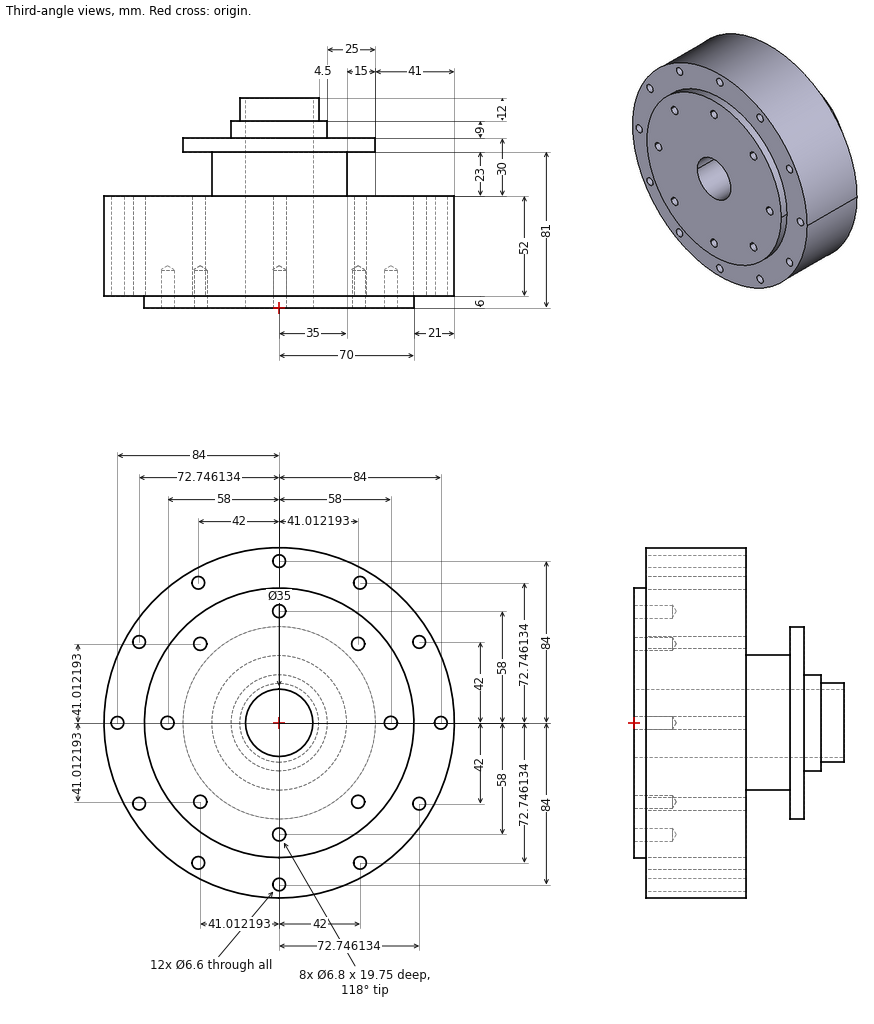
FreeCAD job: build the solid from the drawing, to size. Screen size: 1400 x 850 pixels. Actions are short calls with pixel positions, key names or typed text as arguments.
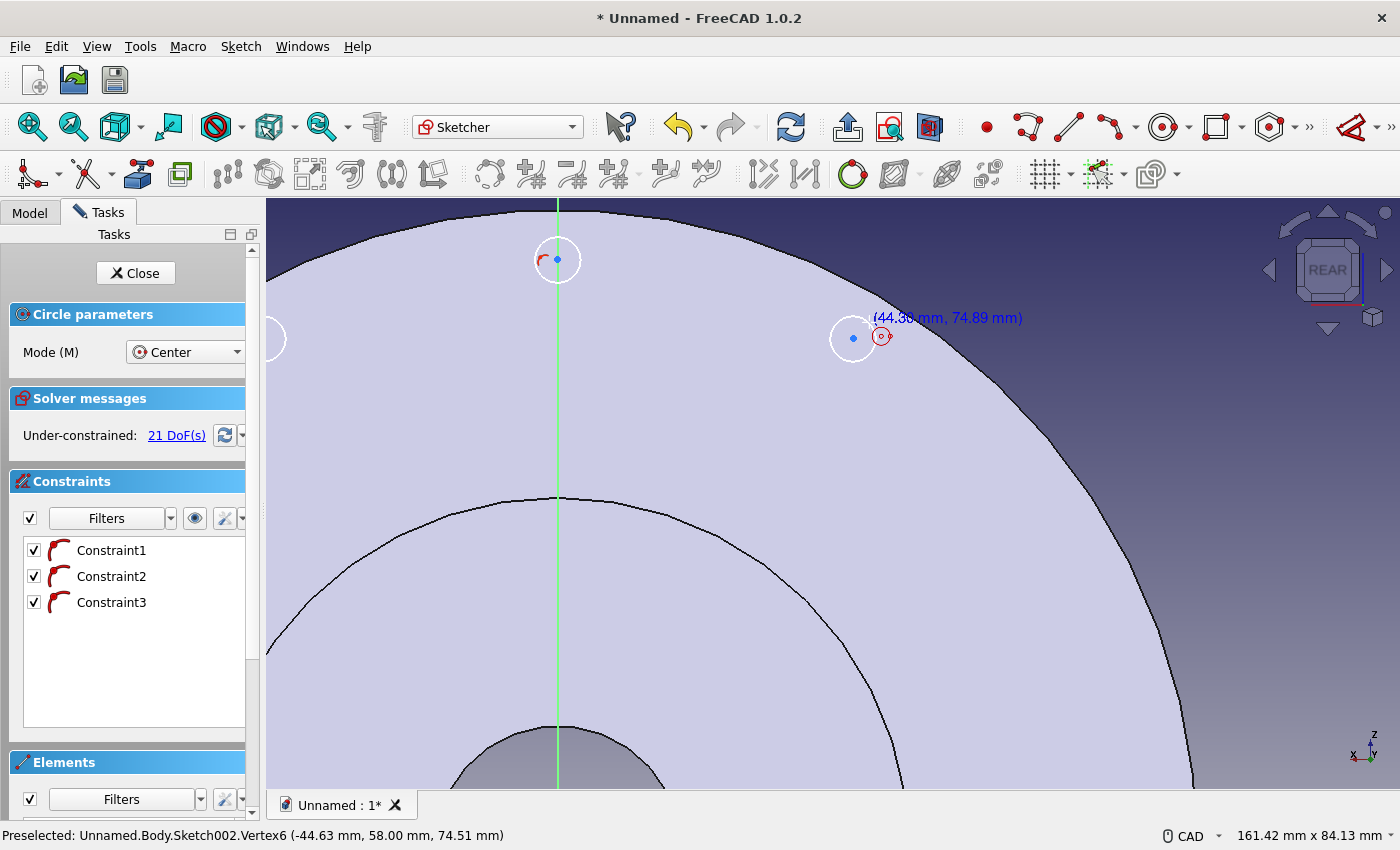
click(1069, 554)
click(1085, 538)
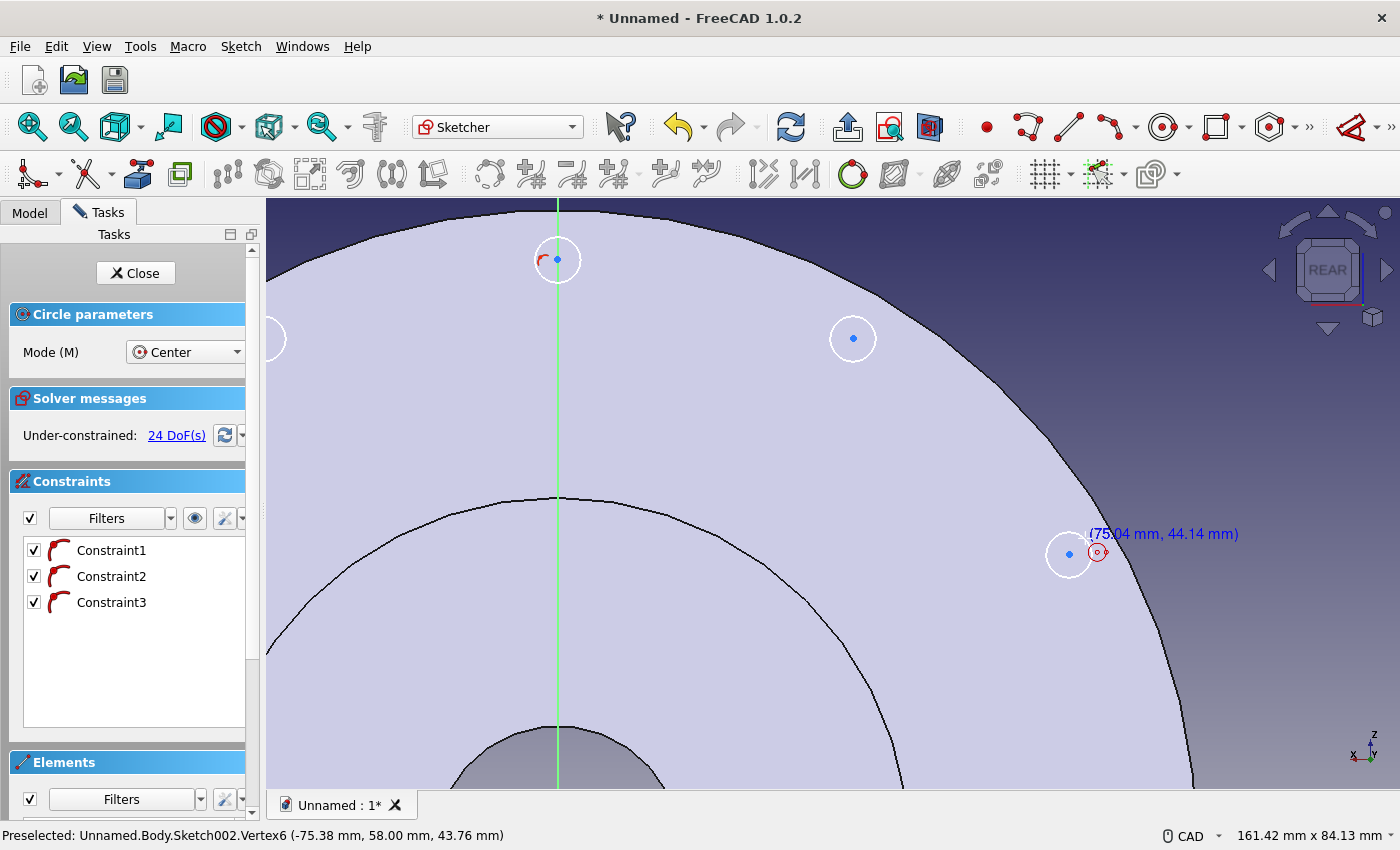
scroll(854, 340, down, 6)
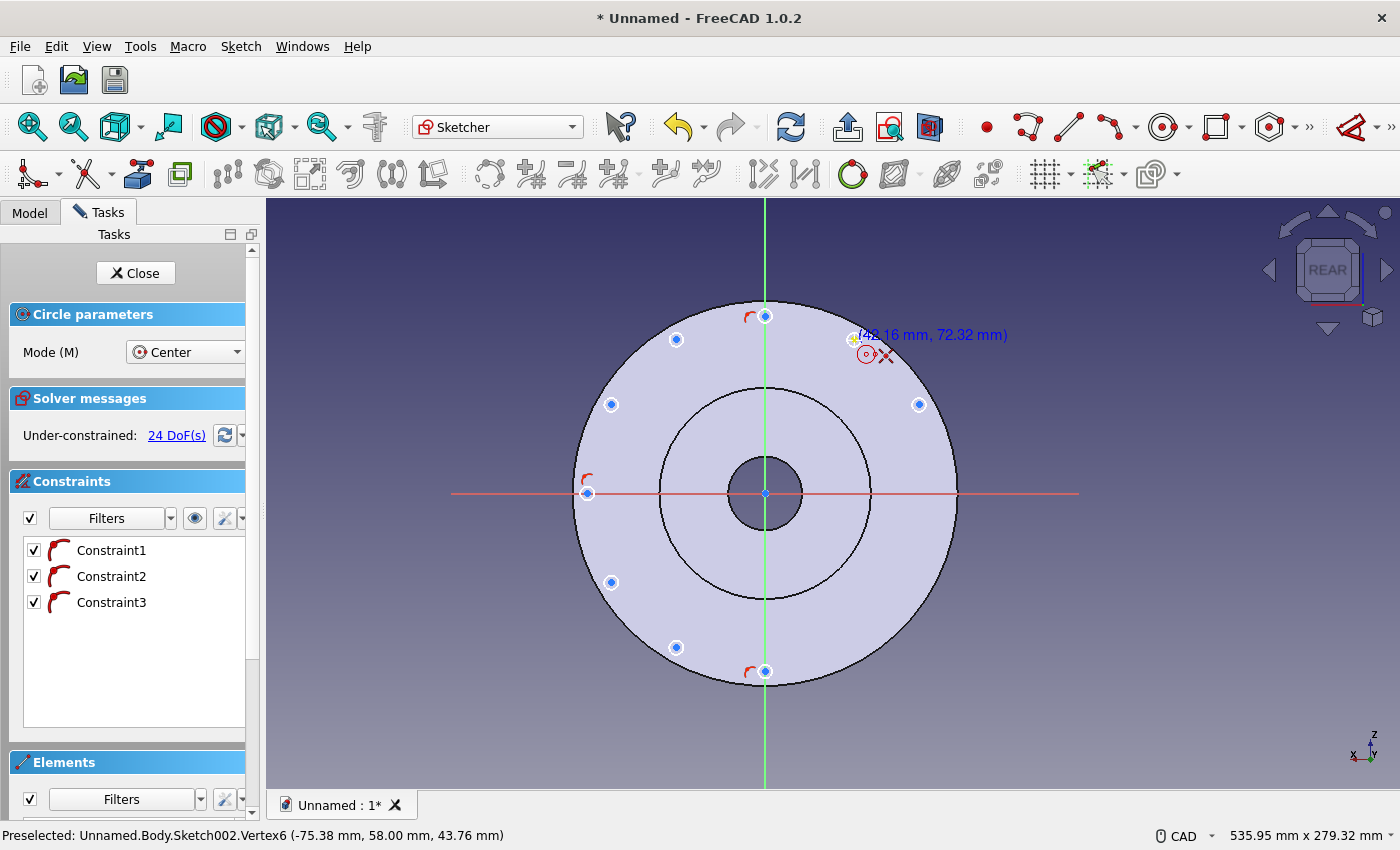
scroll(943, 494, up, 6)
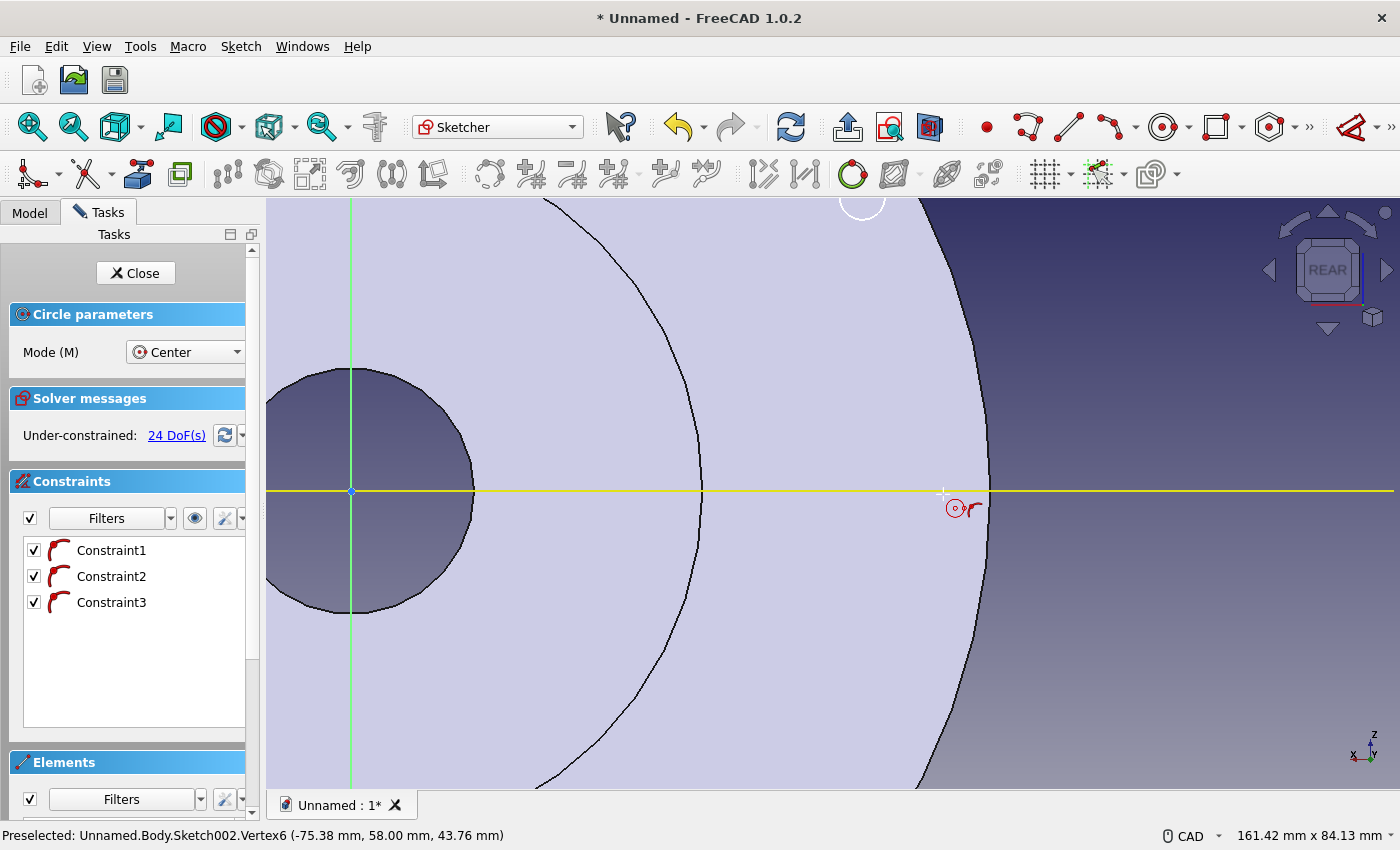
click(941, 491)
click(958, 475)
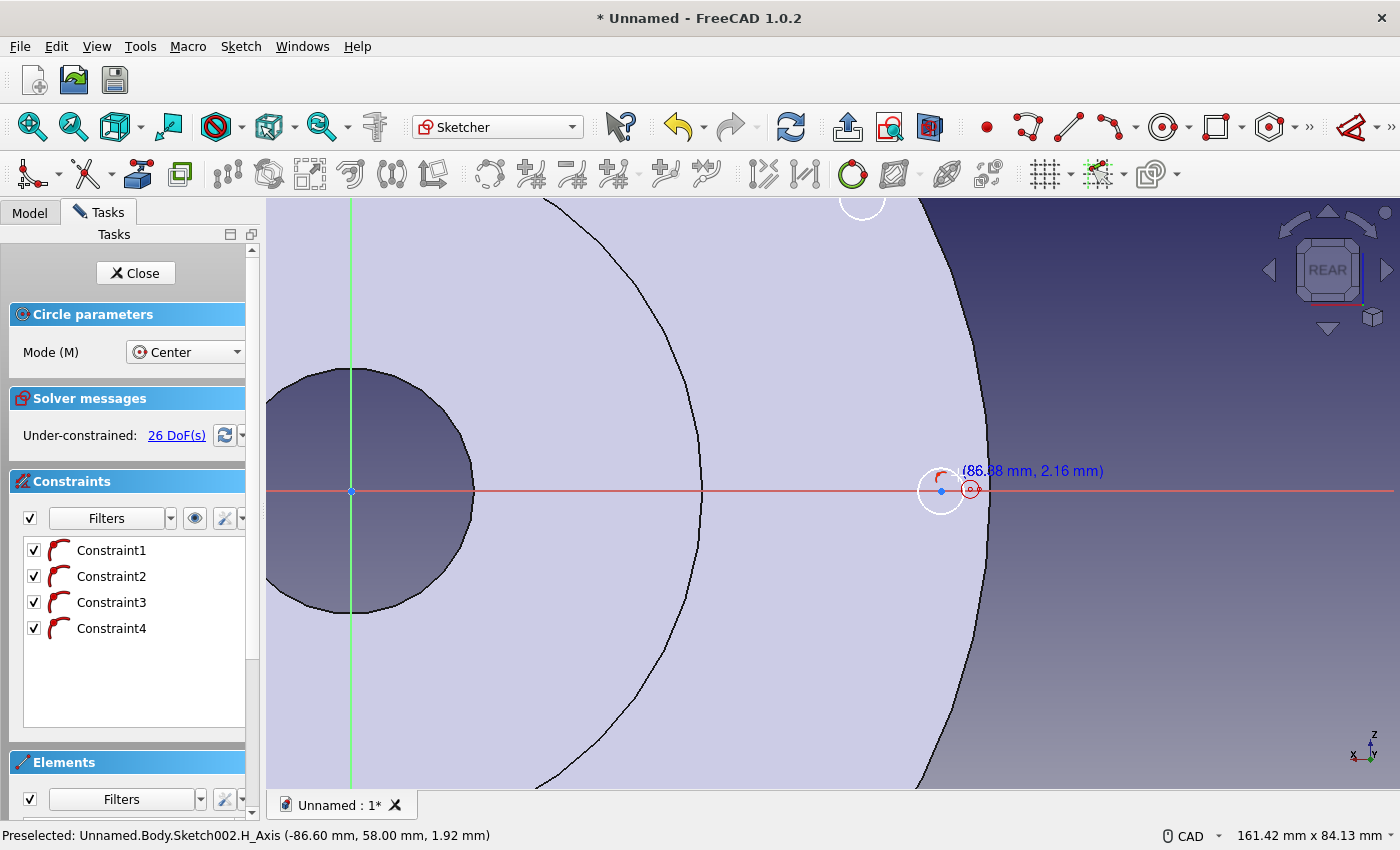
scroll(943, 495, down, 6)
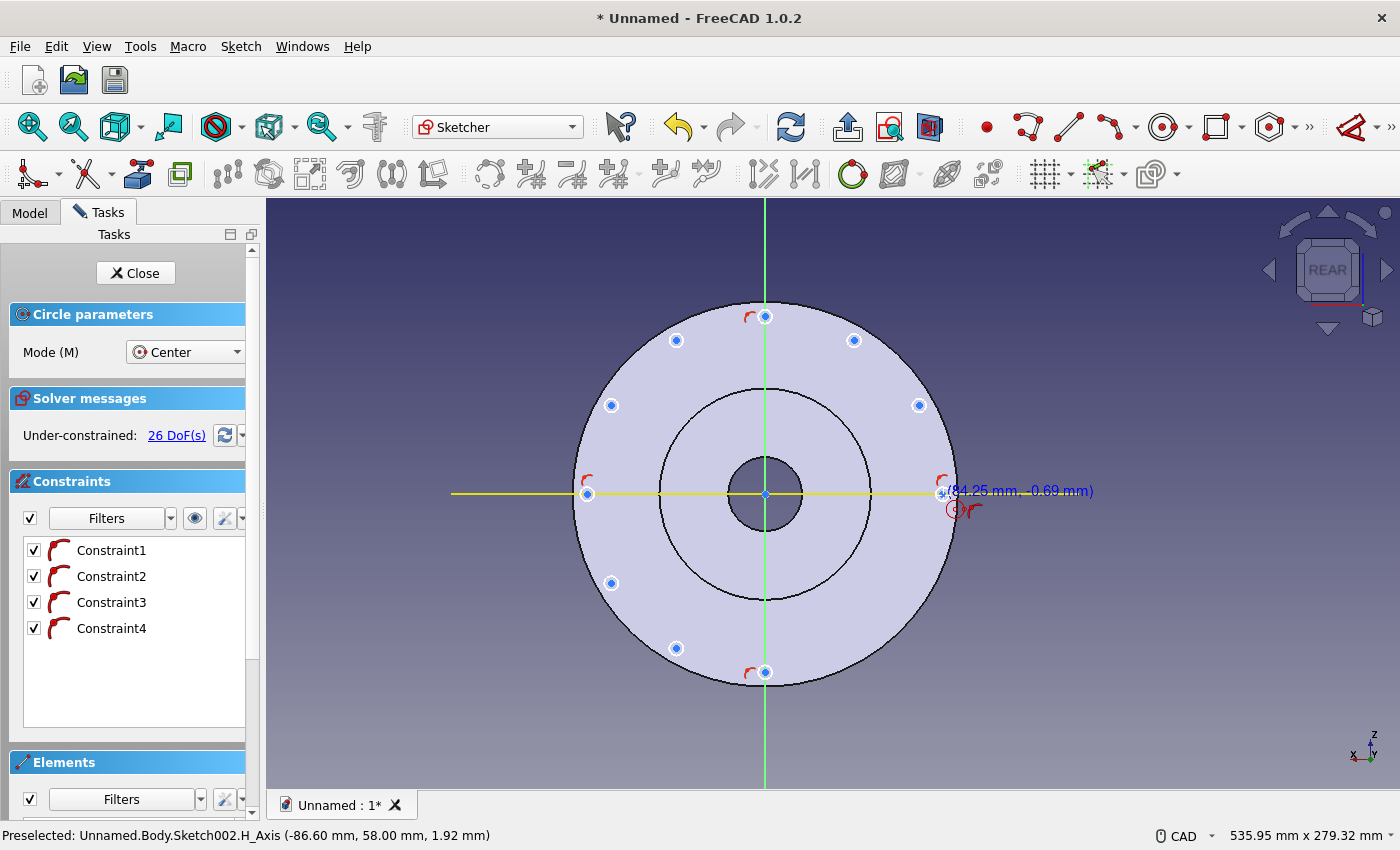
scroll(919, 583, up, 6)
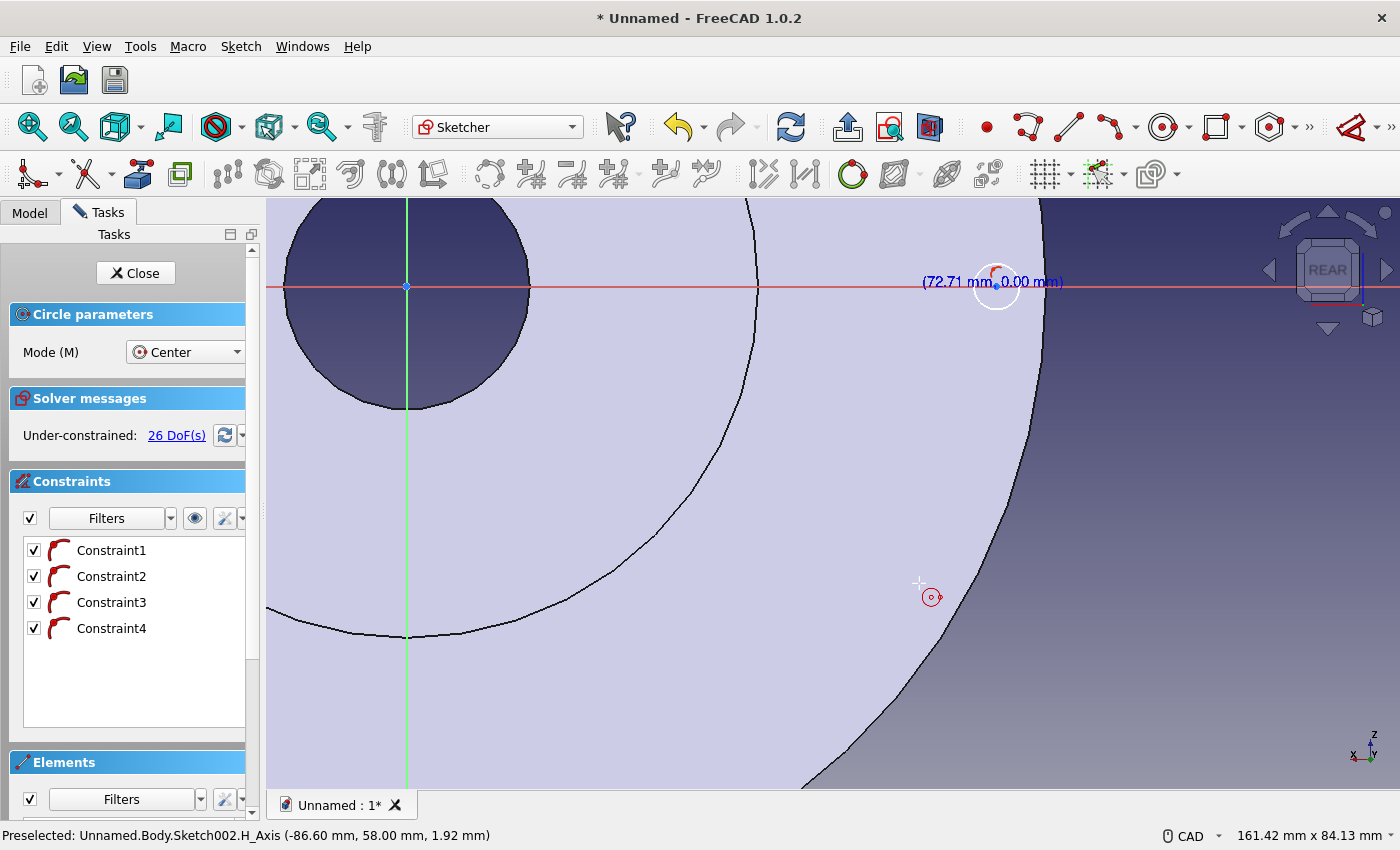
click(918, 582)
click(934, 565)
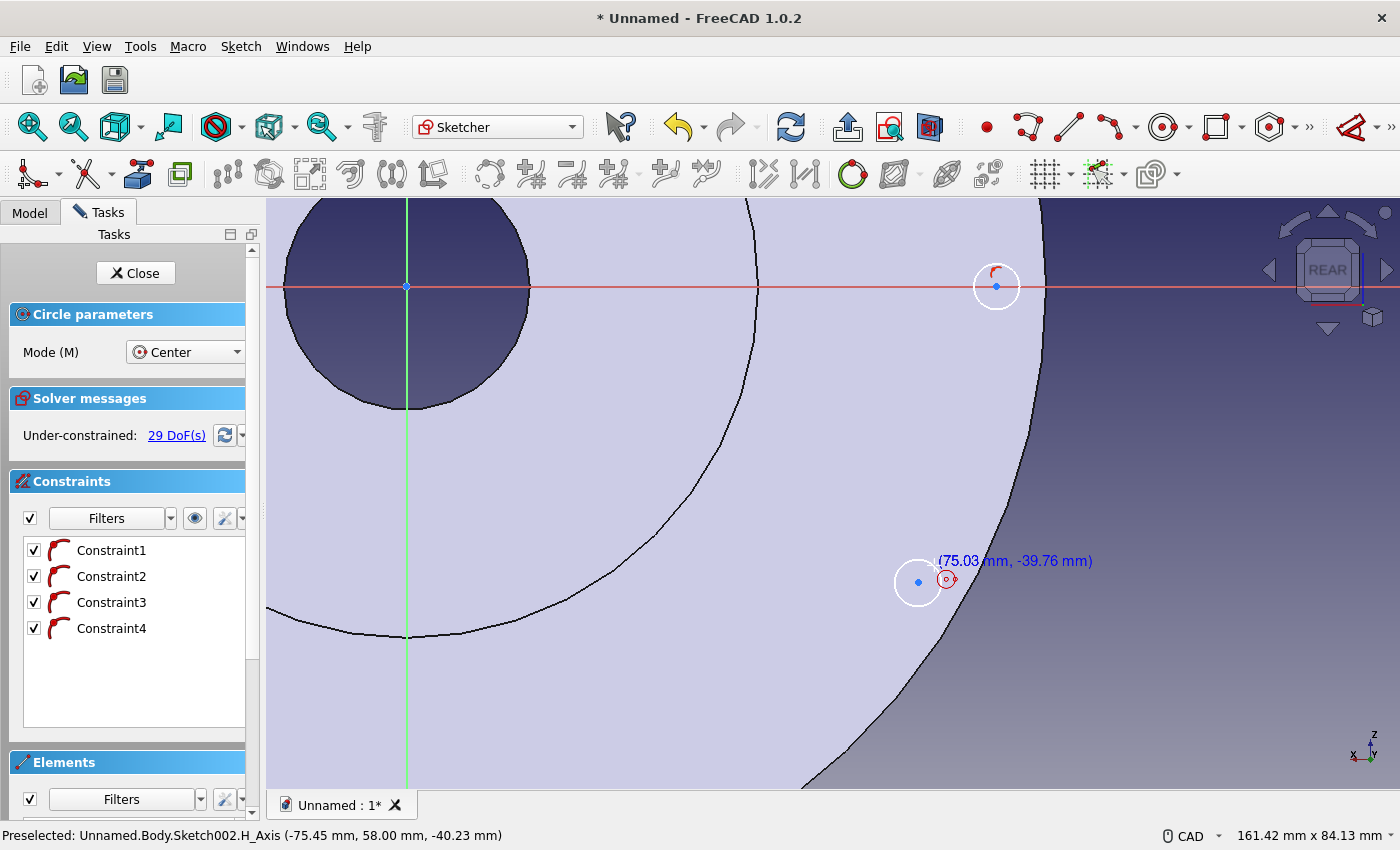
scroll(919, 583, down, 6)